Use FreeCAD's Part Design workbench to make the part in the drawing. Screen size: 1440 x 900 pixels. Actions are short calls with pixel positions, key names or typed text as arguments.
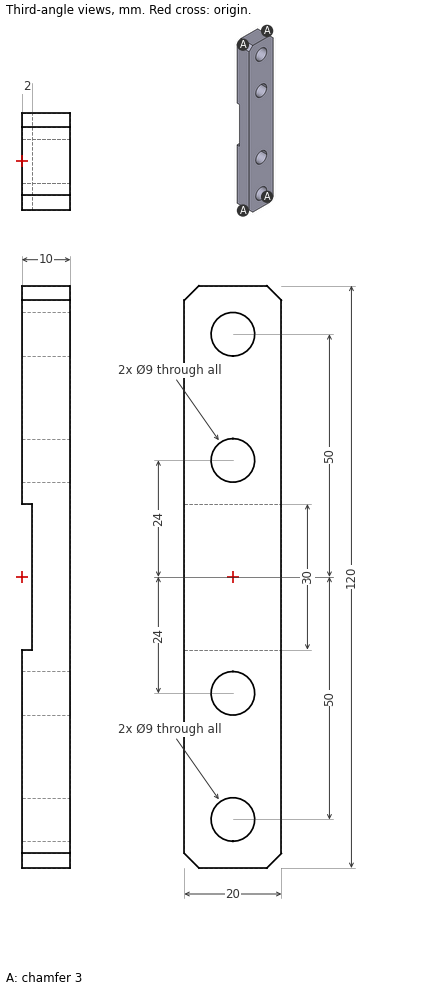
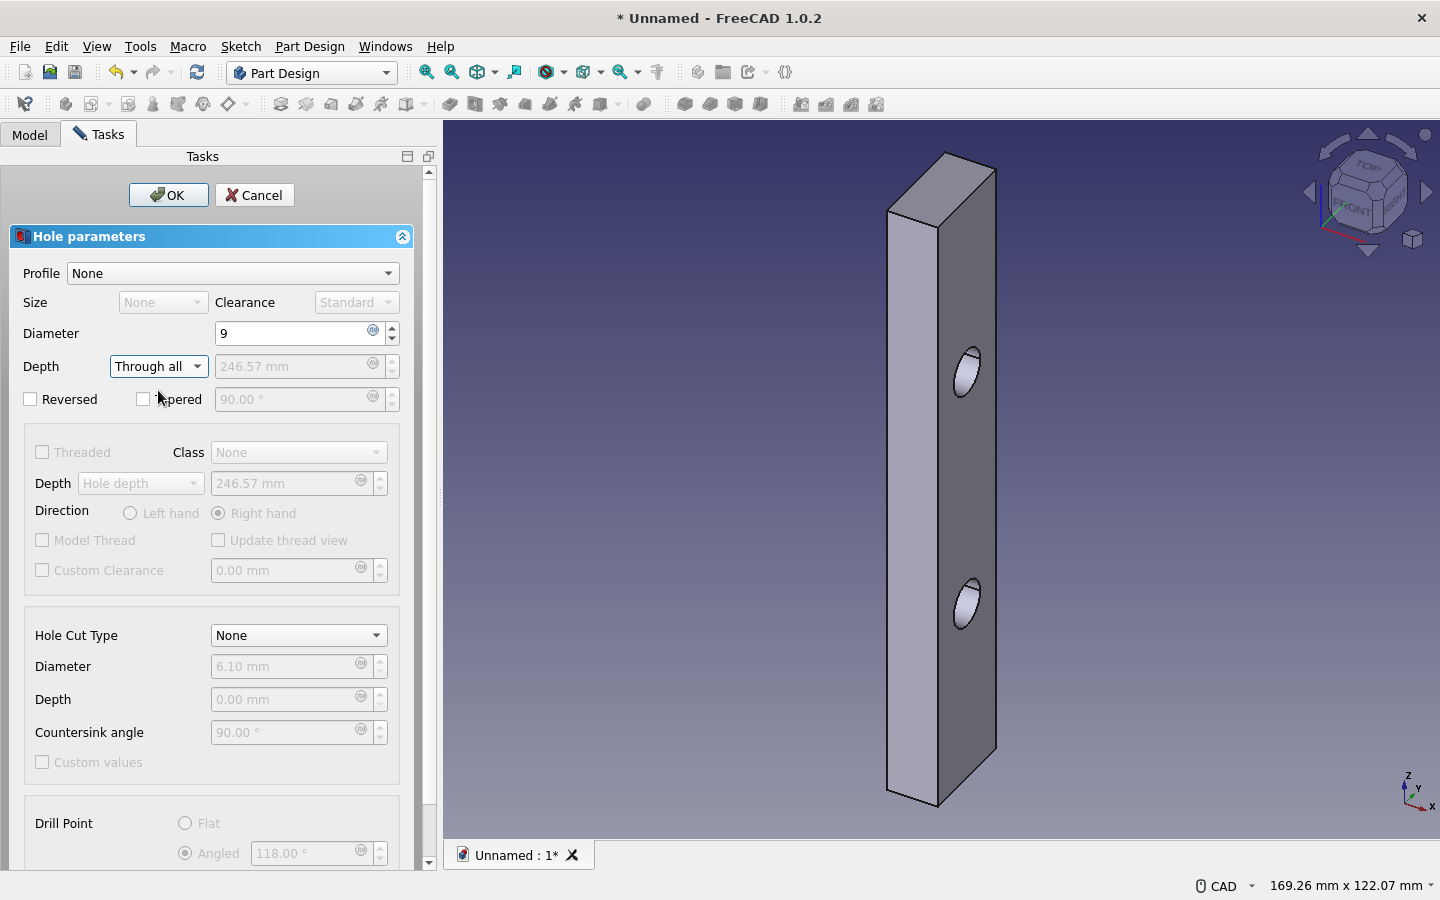
click(169, 195)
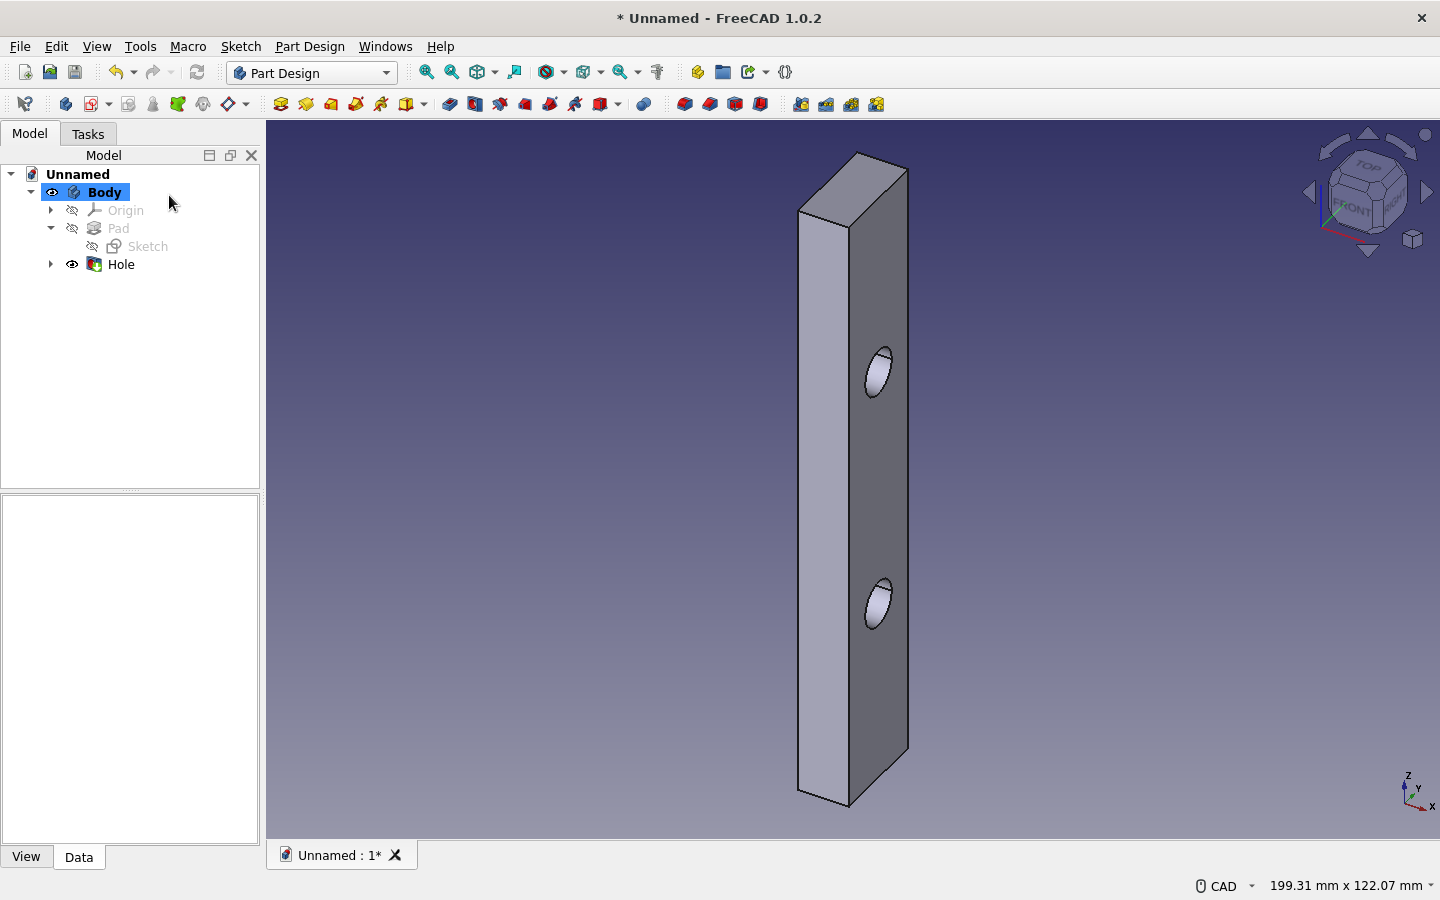
click(90, 104)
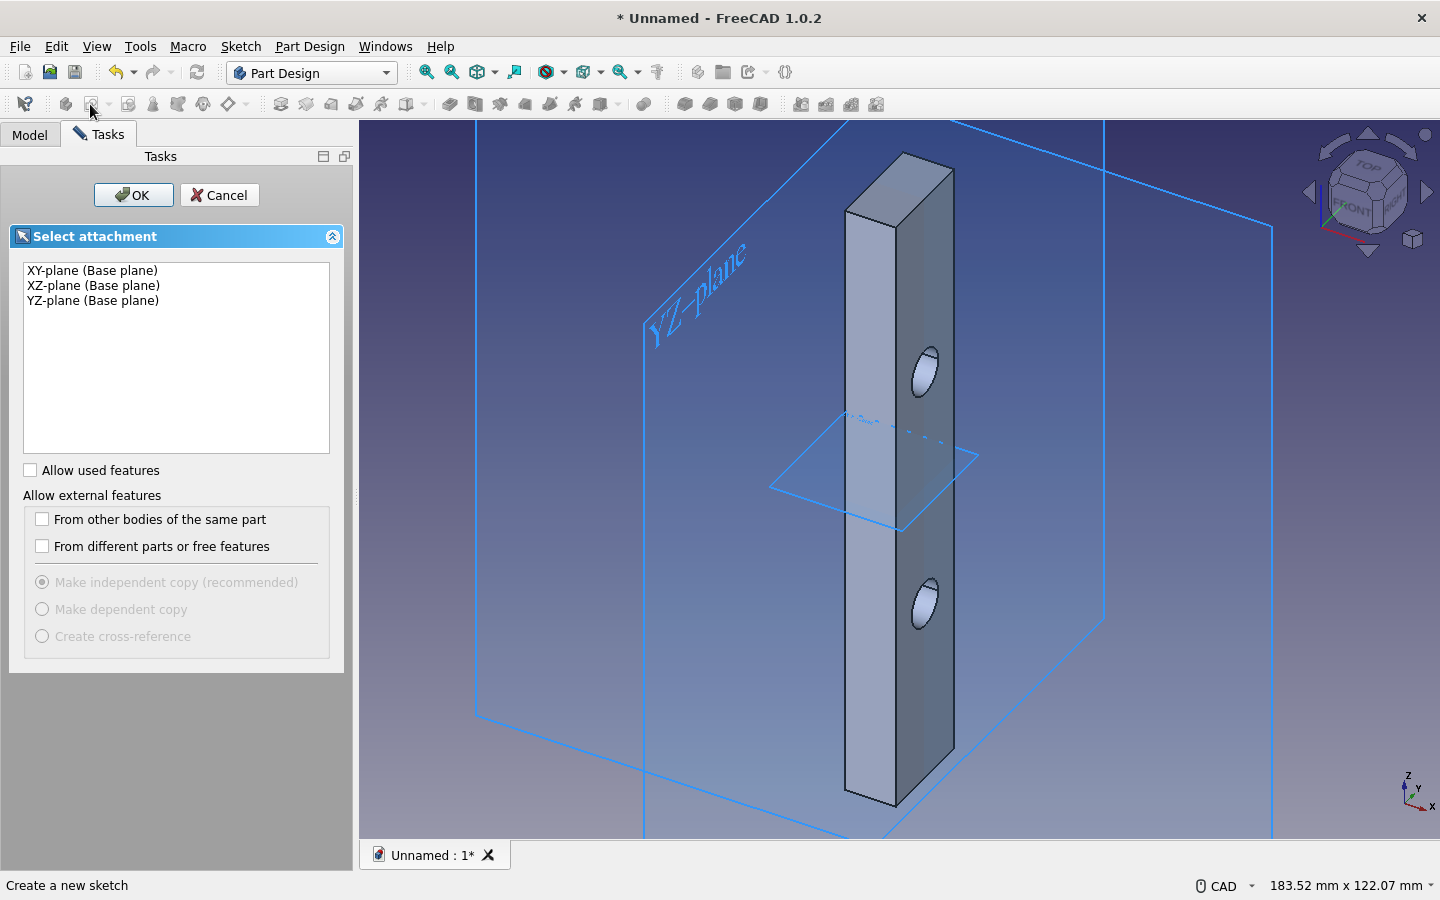
click(84, 300)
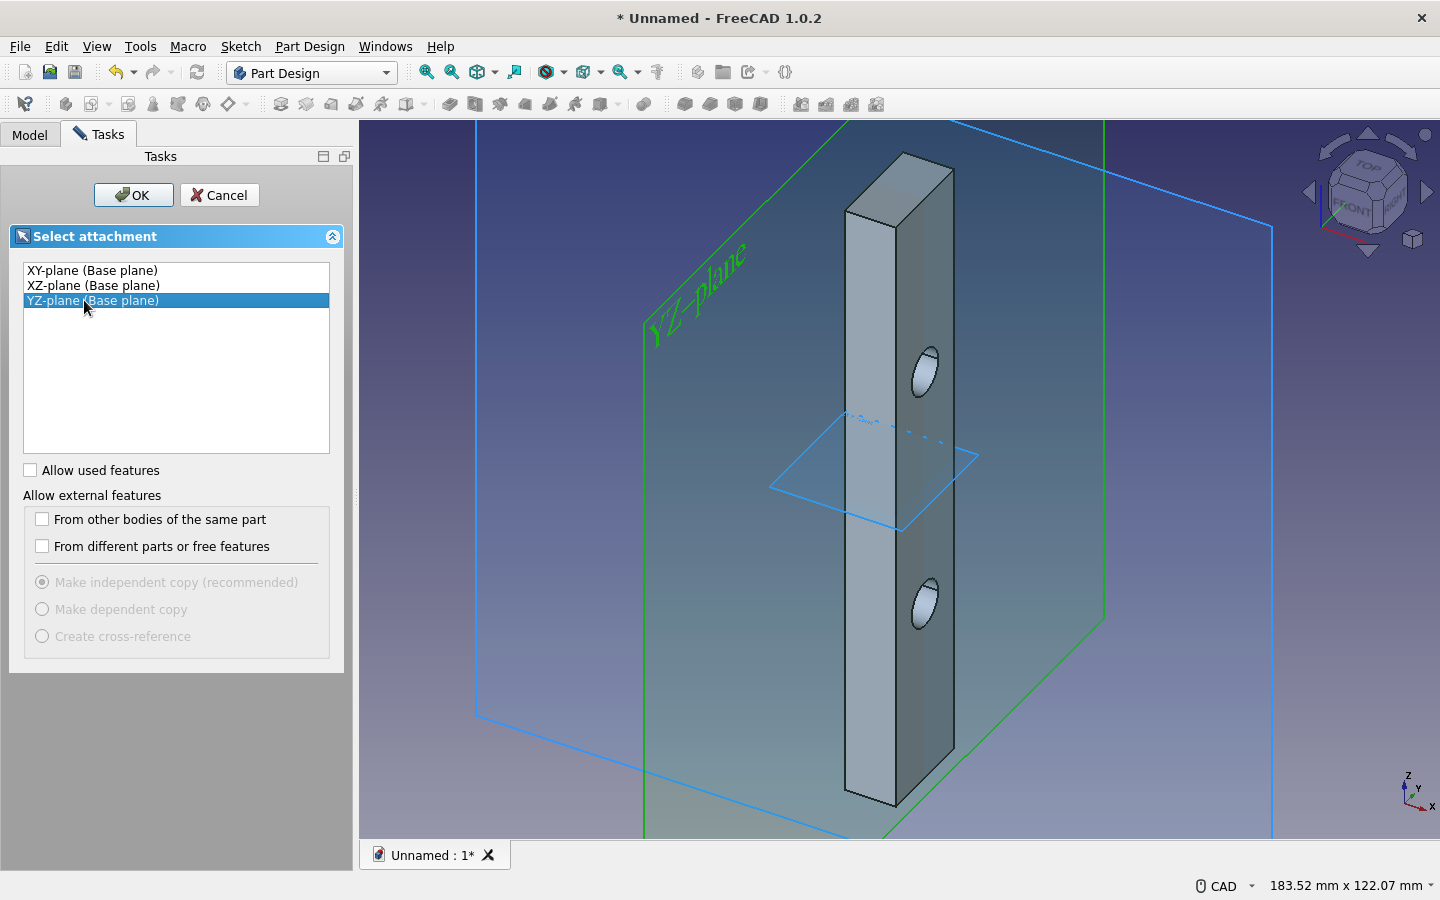
click(134, 195)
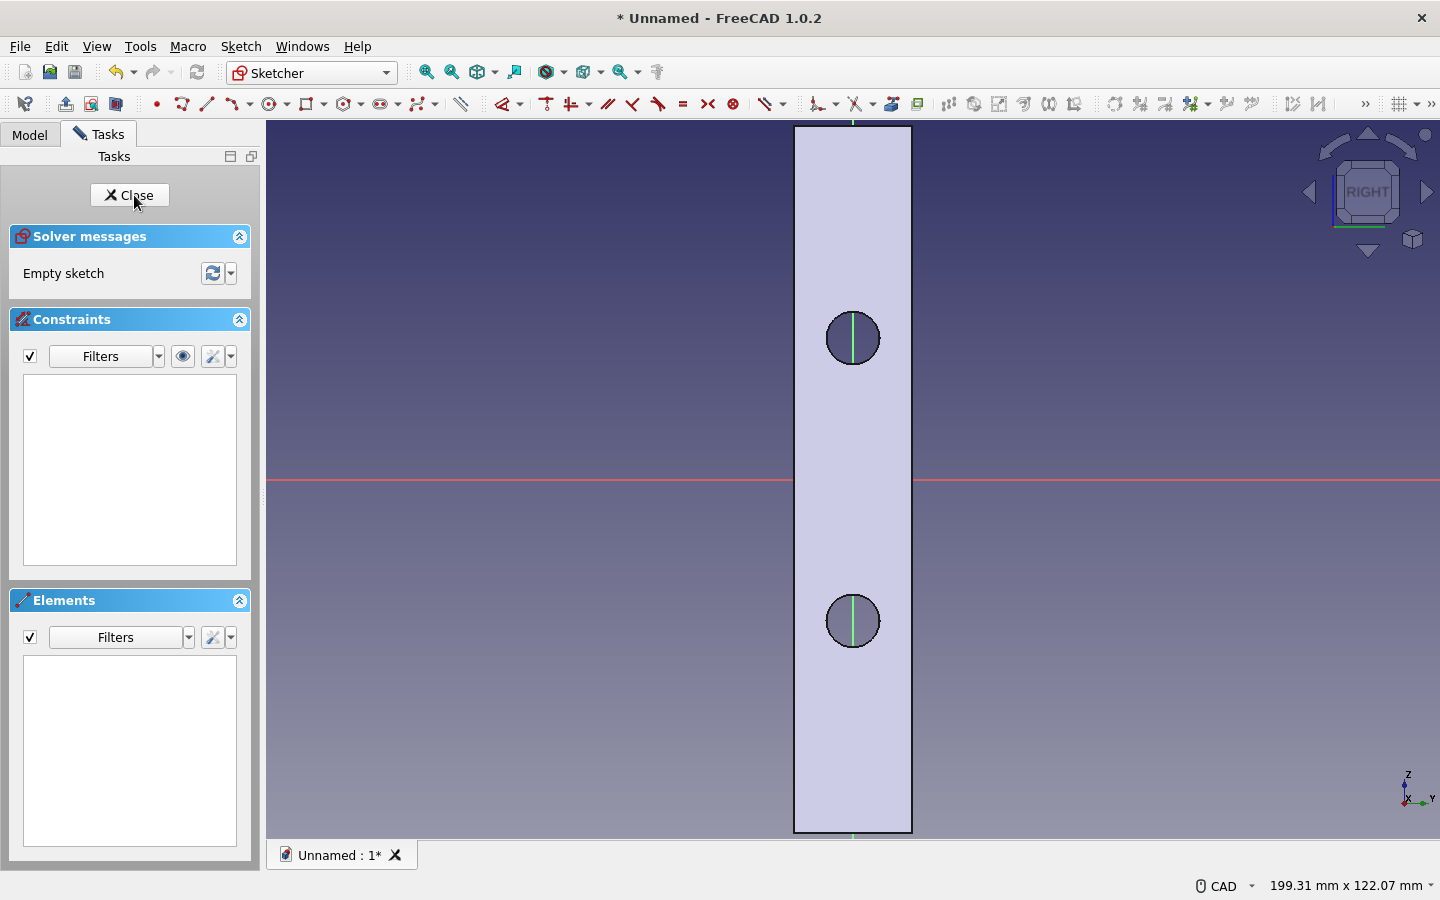
key(q)
key(s)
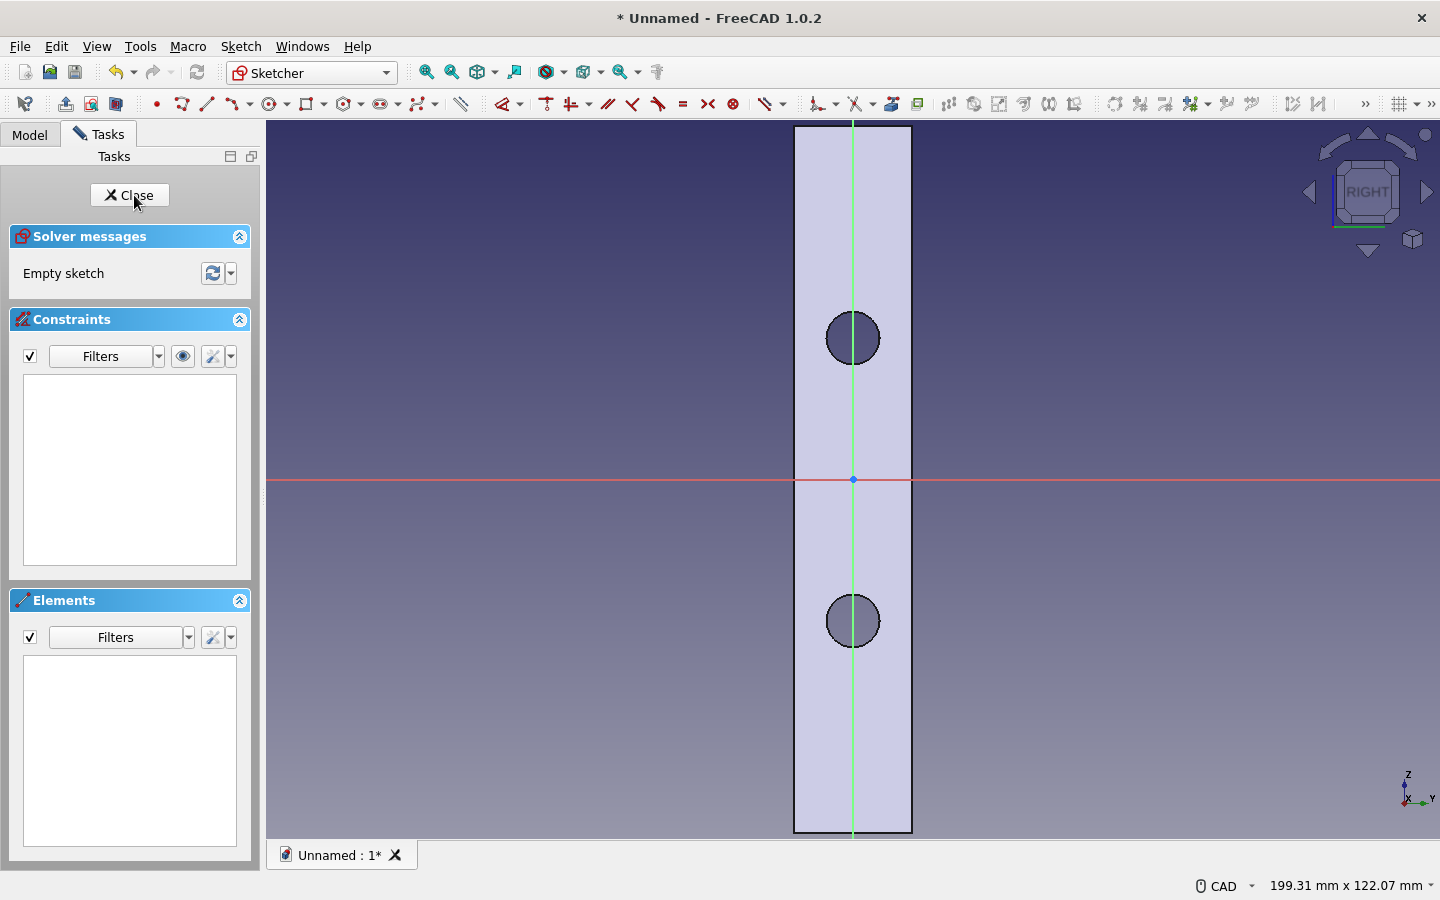
scroll(645, 480, down, 2)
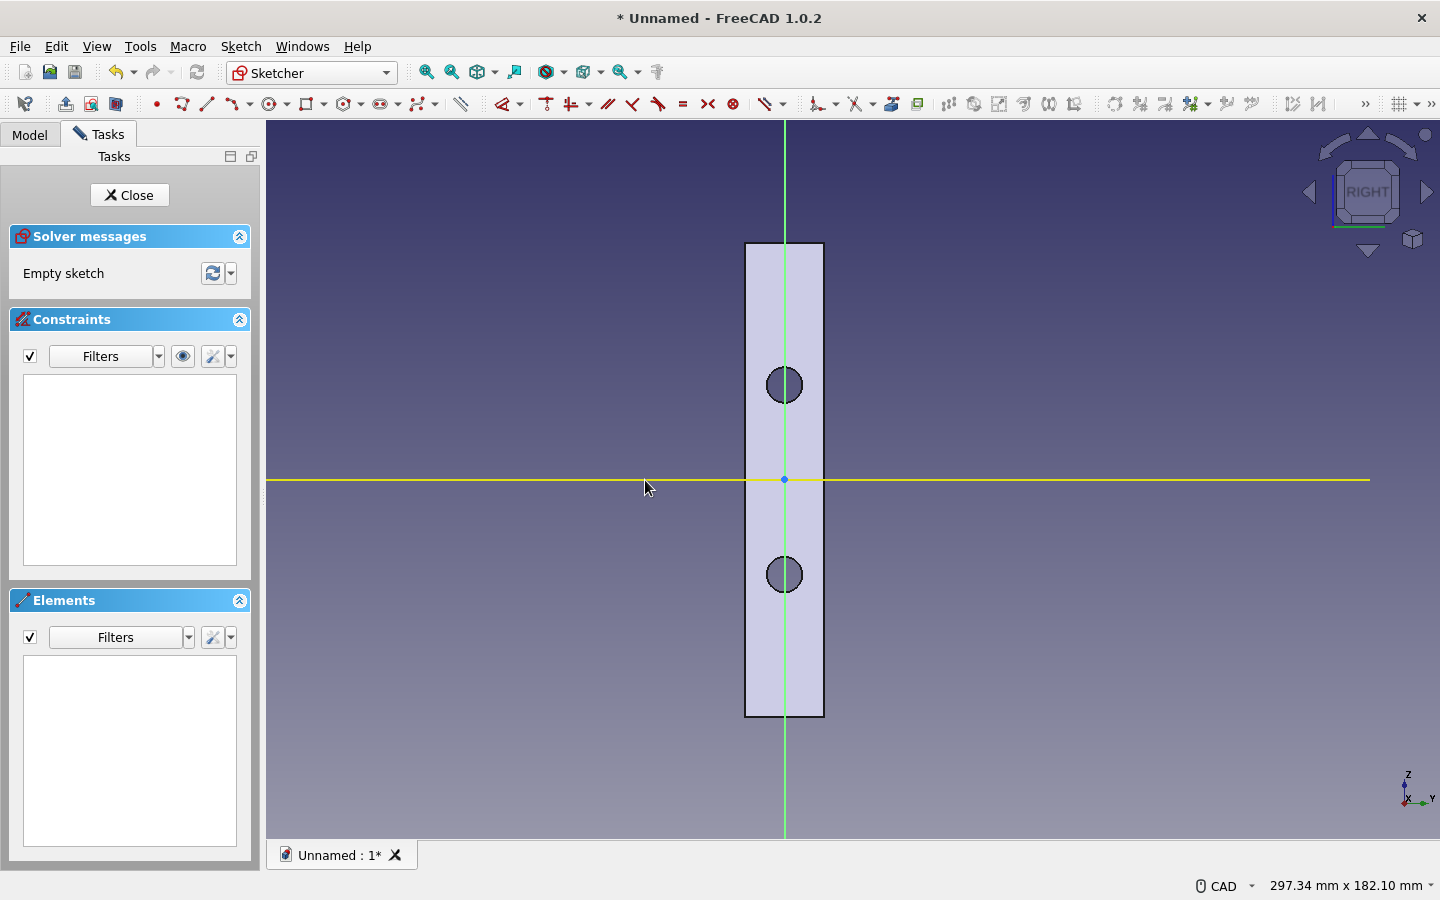
key(g)
key(c)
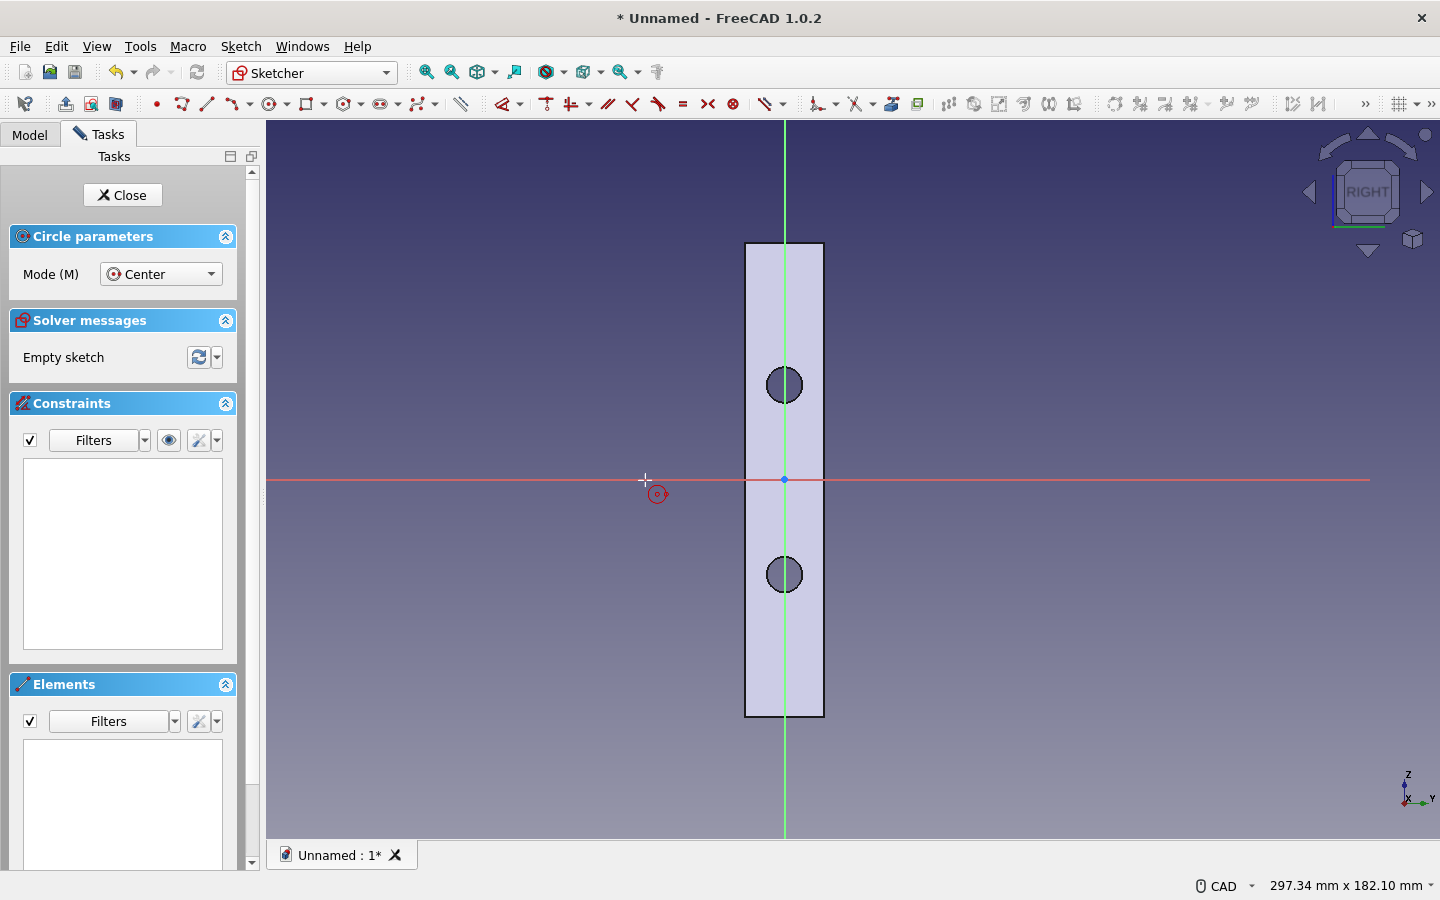
scroll(785, 677, up, 2)